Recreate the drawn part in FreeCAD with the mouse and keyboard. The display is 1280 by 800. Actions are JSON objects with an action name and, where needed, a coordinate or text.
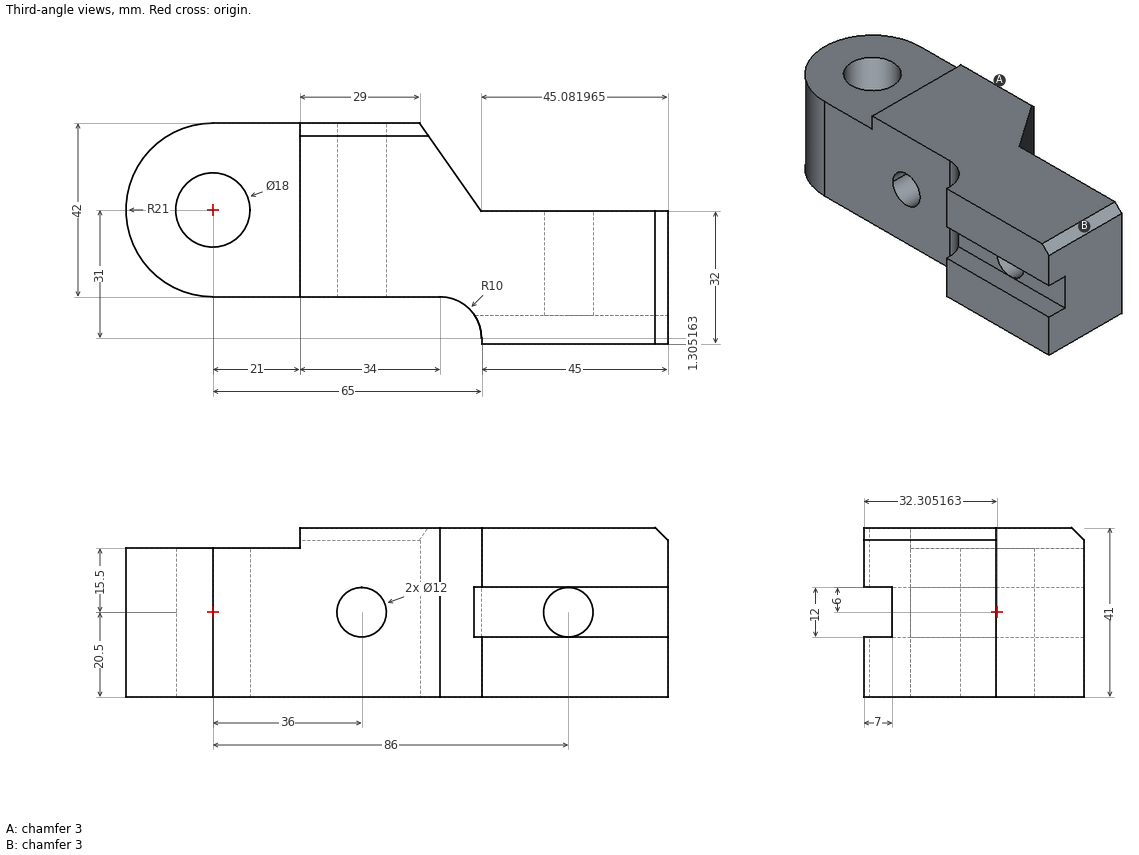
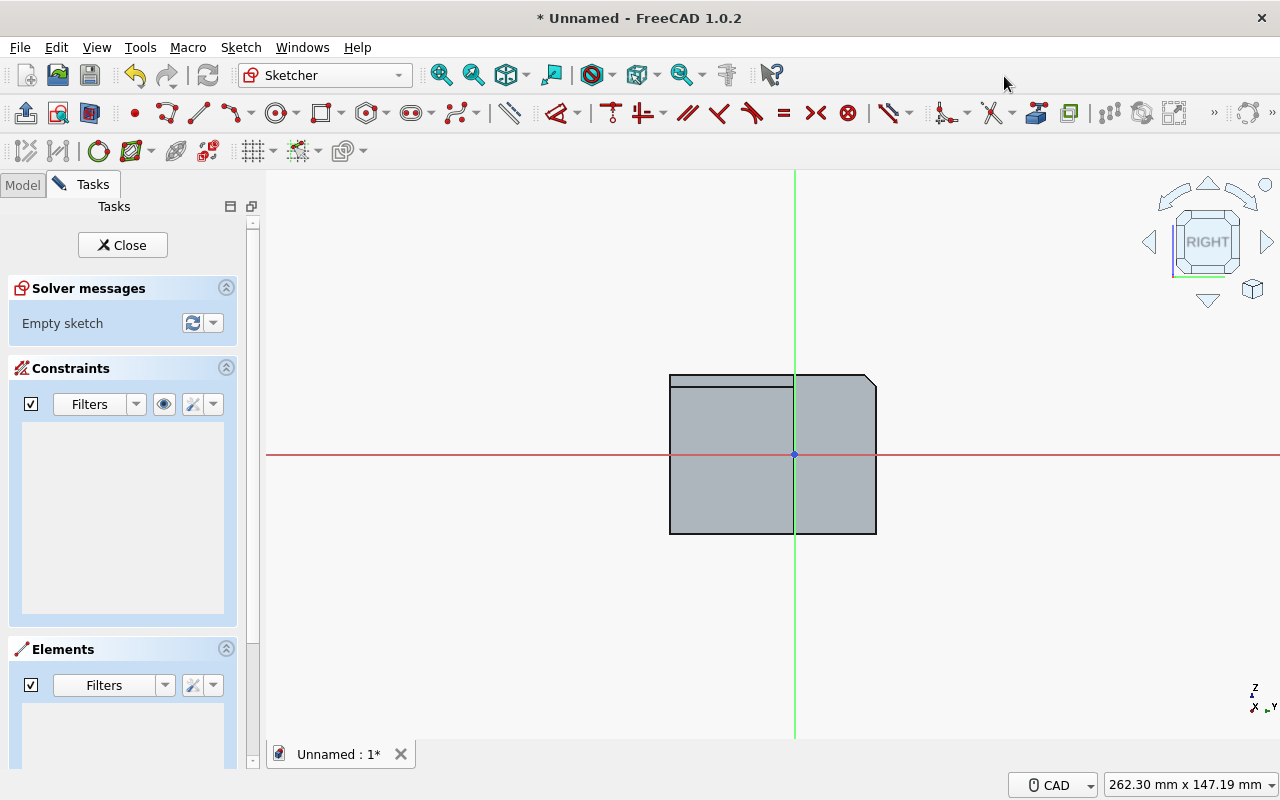
{"action": "scroll", "coordinate": [680, 454], "scroll_direction": "up", "scroll_amount": 10}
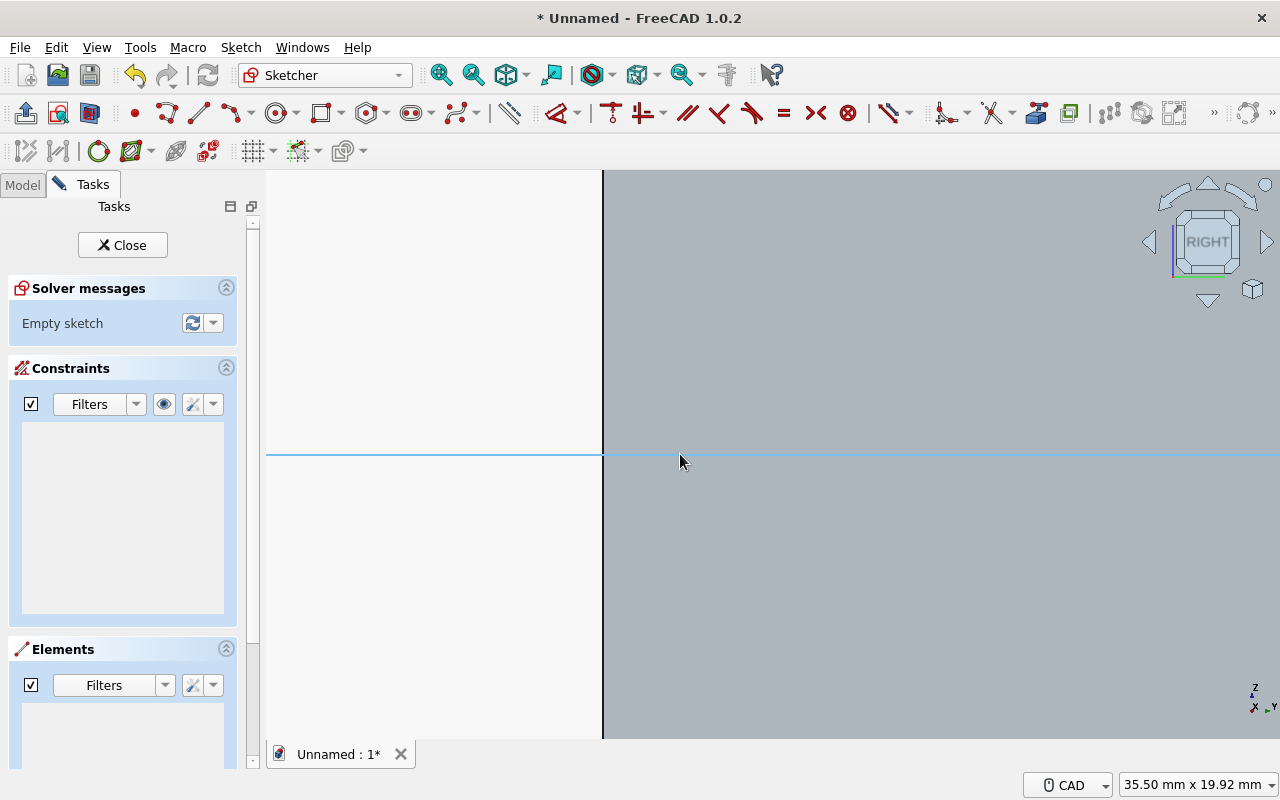
{"action": "left_click", "coordinate": [322, 114]}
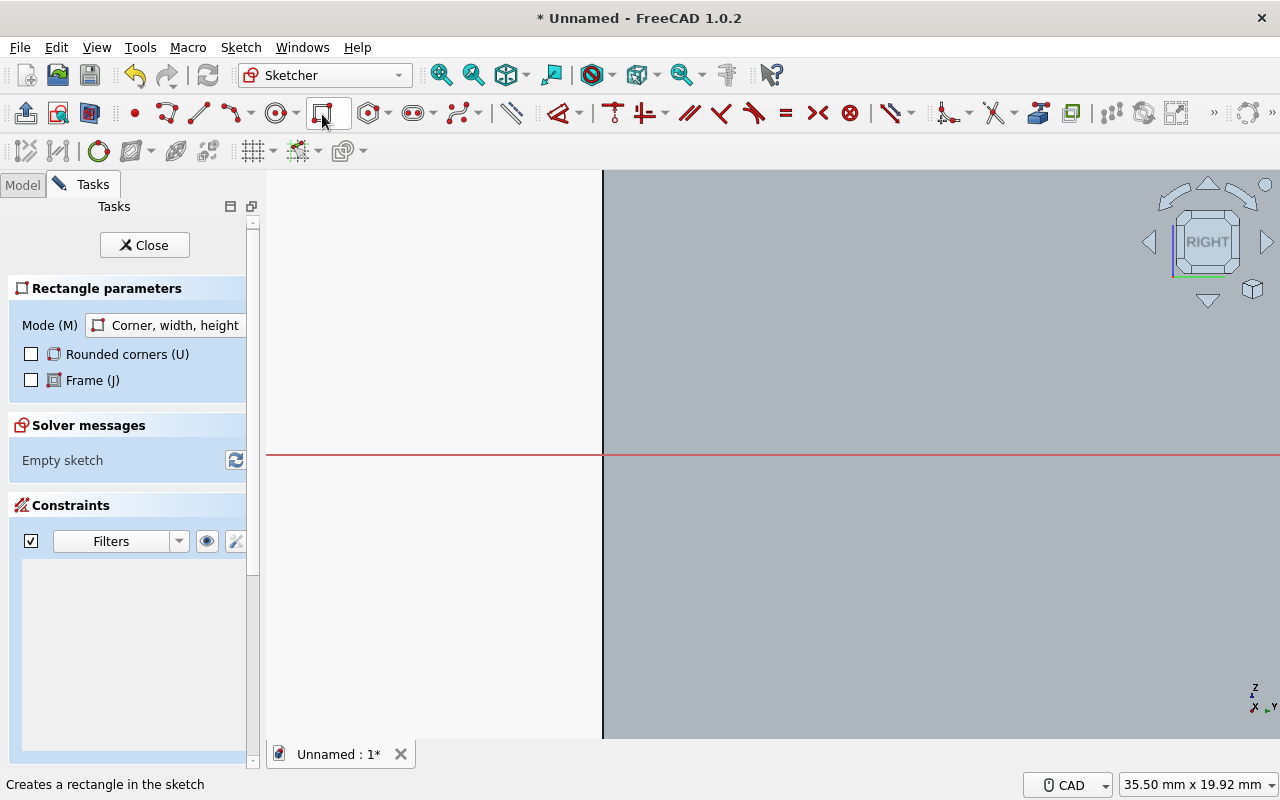
{"action": "left_click", "coordinate": [603, 283]}
{"action": "mouse_move", "coordinate": [803, 626]}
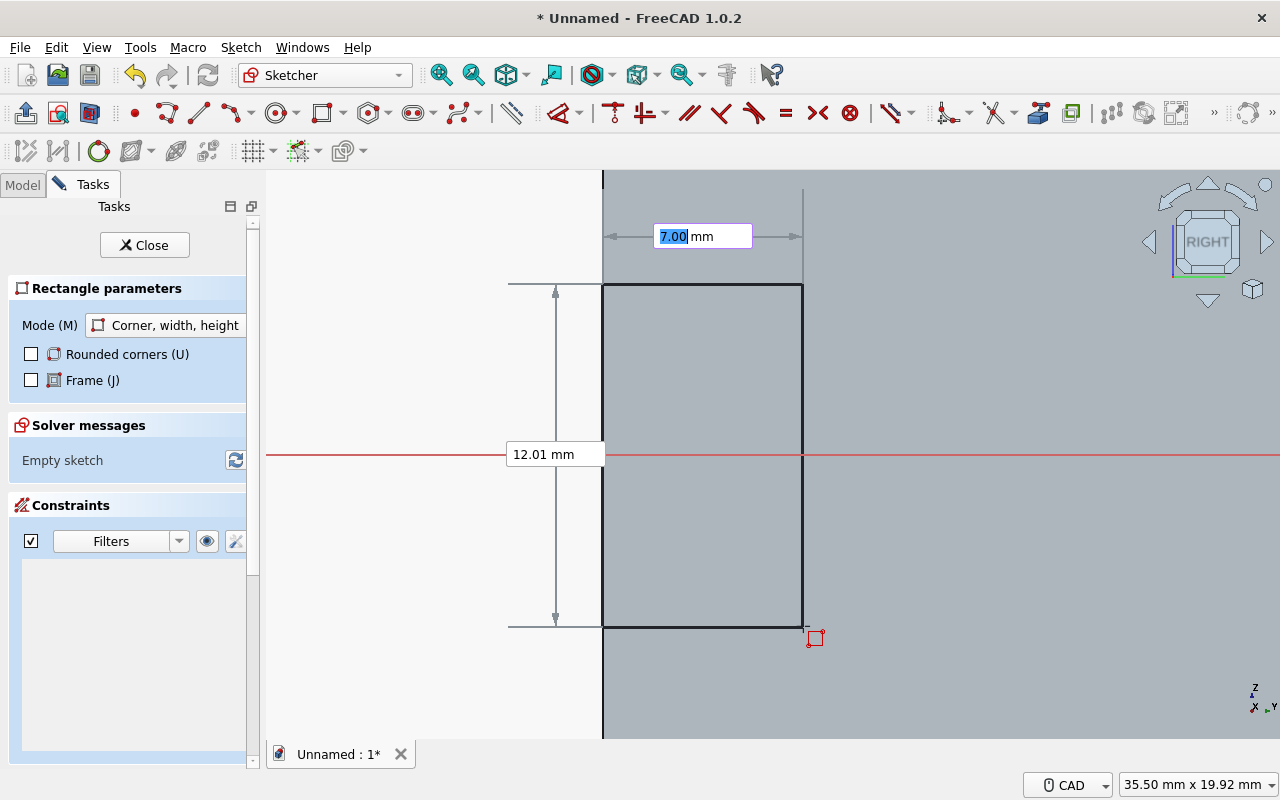
{"action": "type", "text": "7"}
{"action": "key", "text": "Tab"}
{"action": "type", "text": "12"}
{"action": "key", "text": "Return"}
{"action": "key", "text": "Escape"}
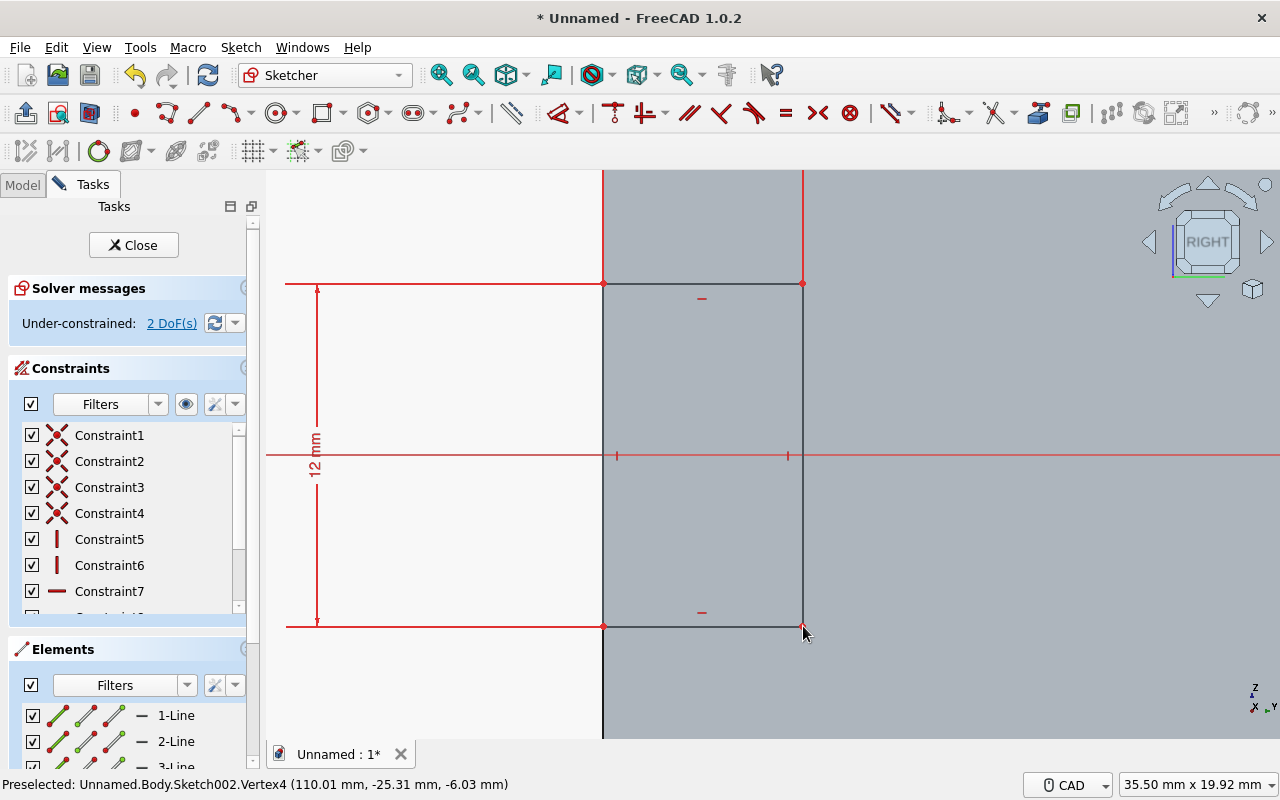
{"action": "left_click", "coordinate": [558, 114]}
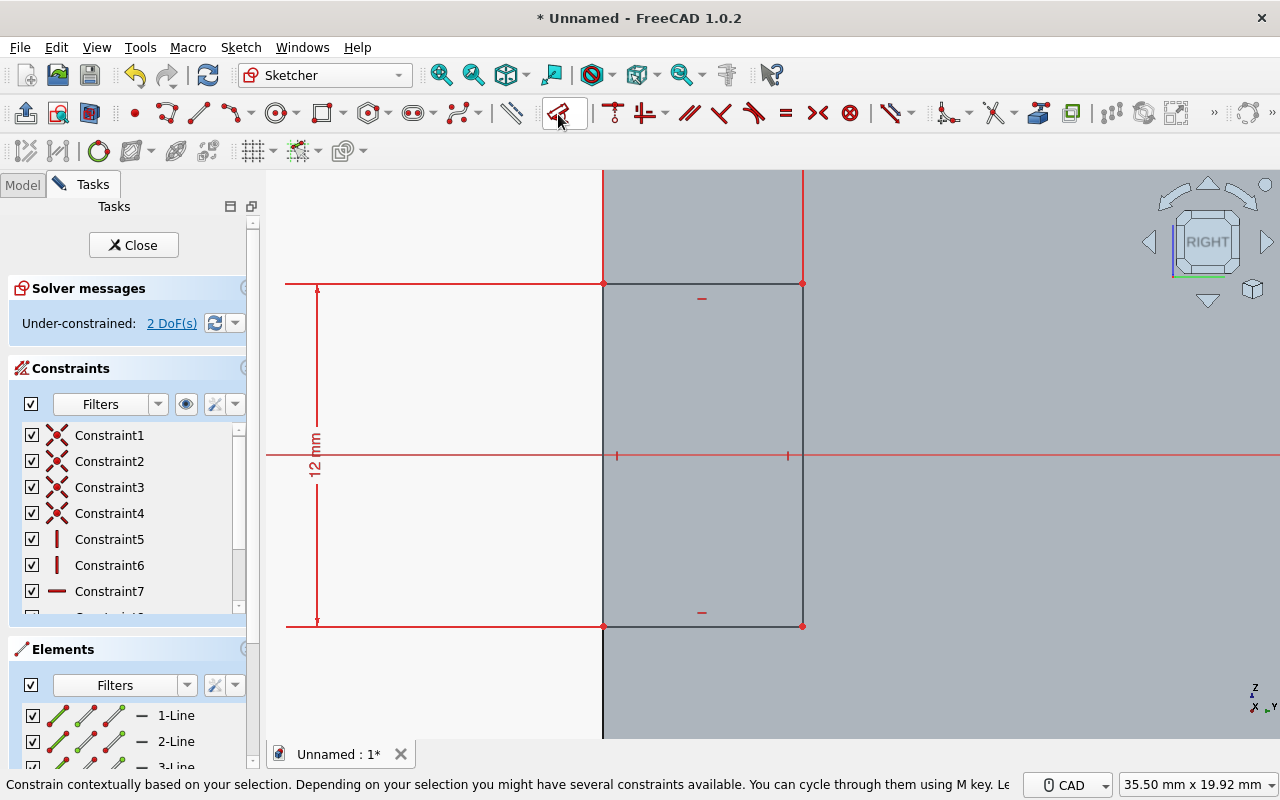
{"action": "left_click", "coordinate": [603, 284]}
{"action": "left_click", "coordinate": [569, 369]}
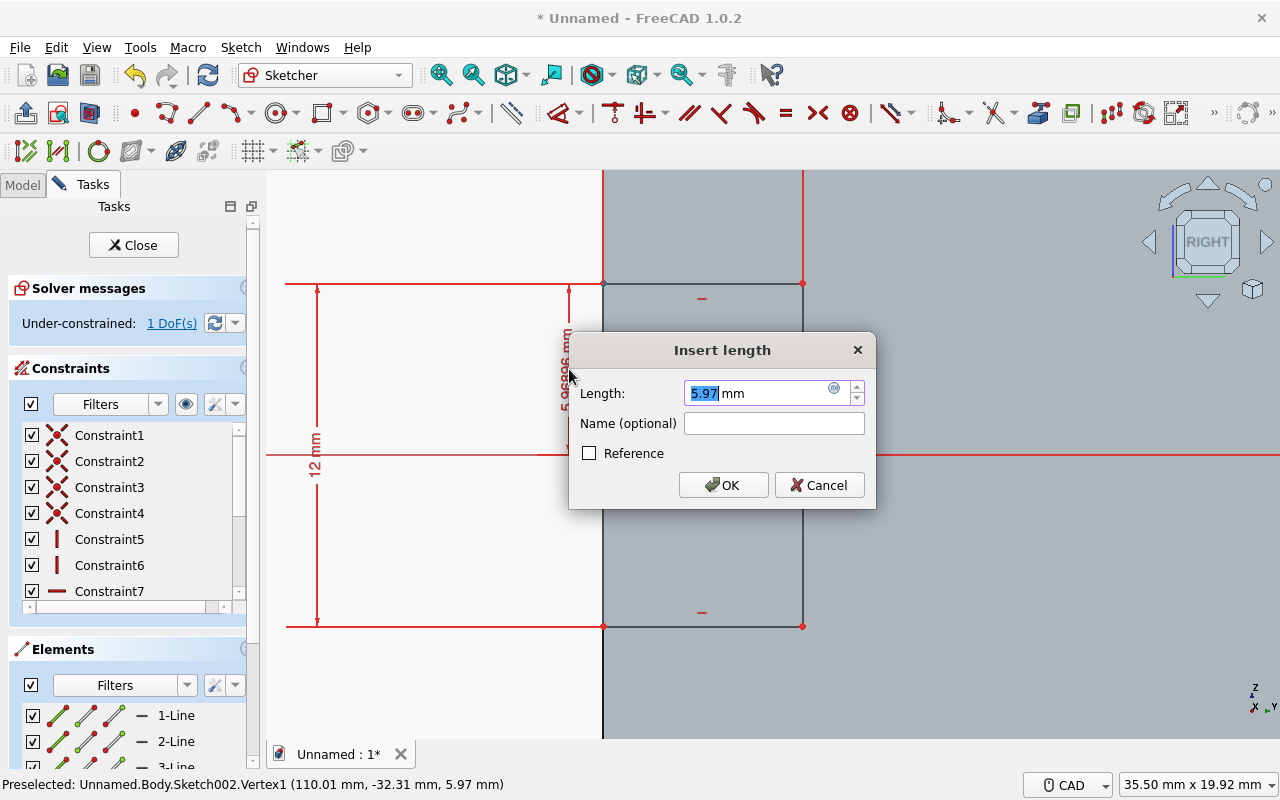
{"action": "type", "text": "6"}
{"action": "key", "text": "Return"}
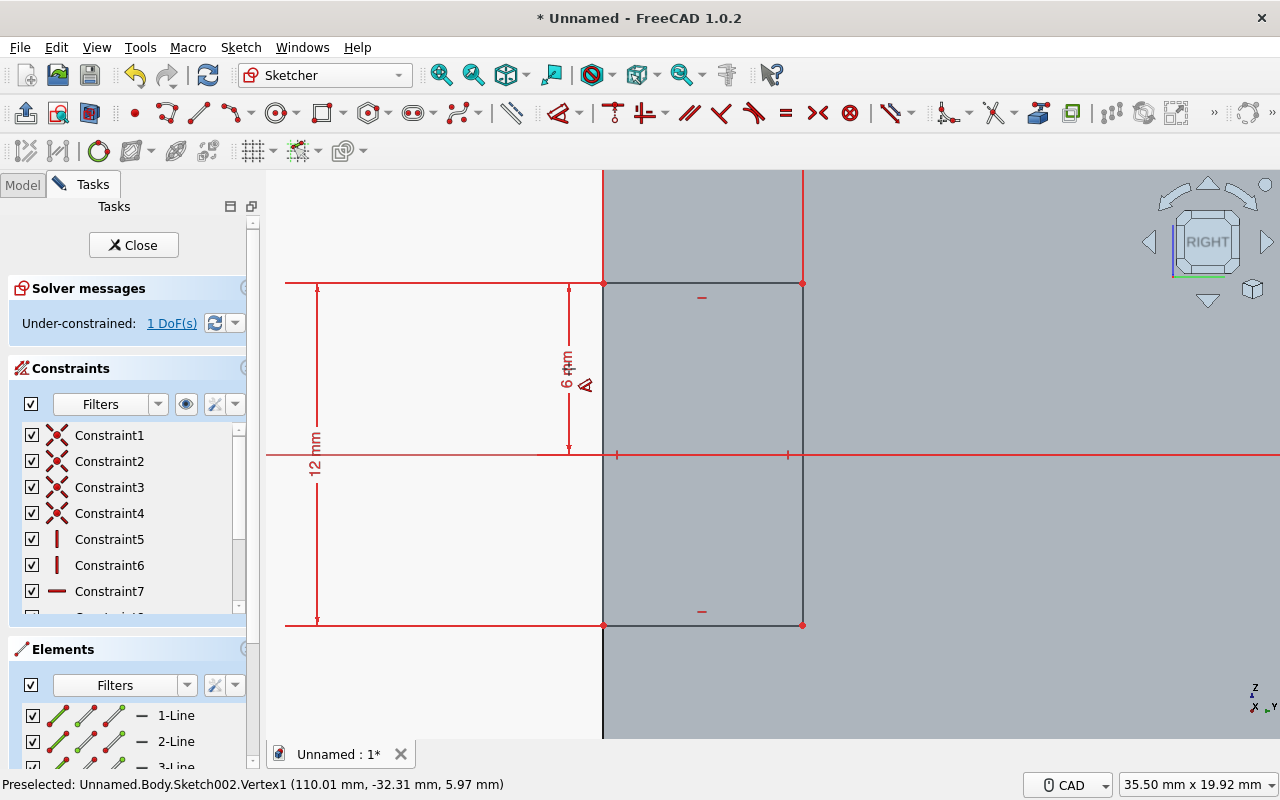
{"action": "left_click", "coordinate": [603, 283]}
{"action": "left_click", "coordinate": [859, 249]}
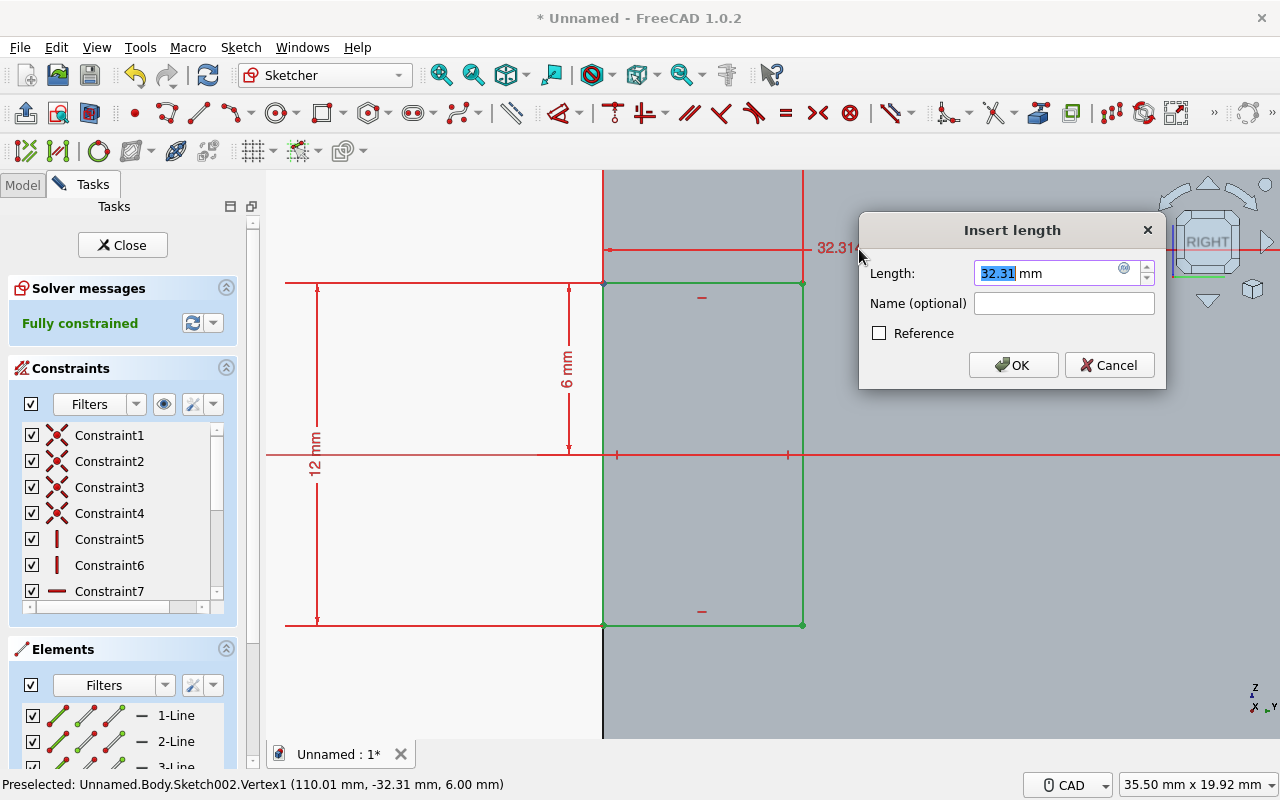
{"action": "type", "text": "32.305163"}
{"action": "key", "text": "Return"}
{"action": "key", "text": "Escape"}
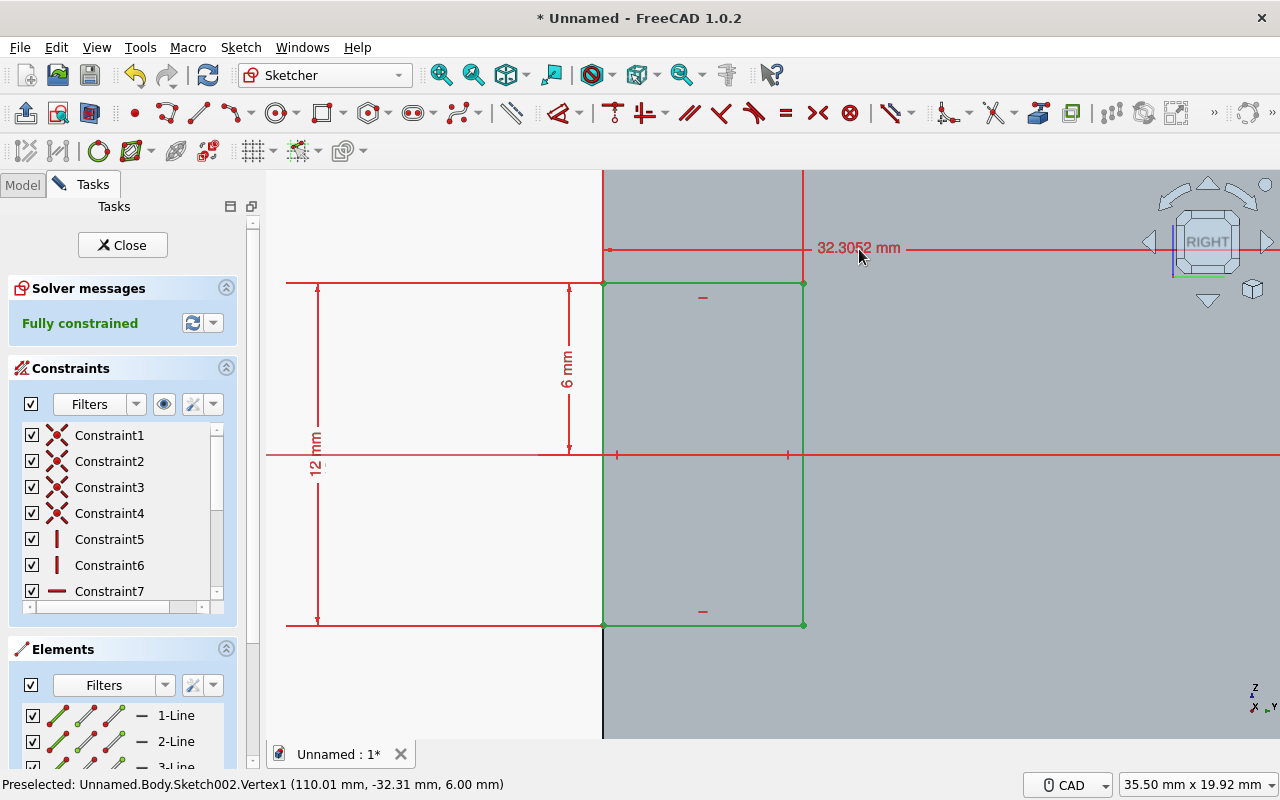
{"action": "left_click", "coordinate": [123, 245]}